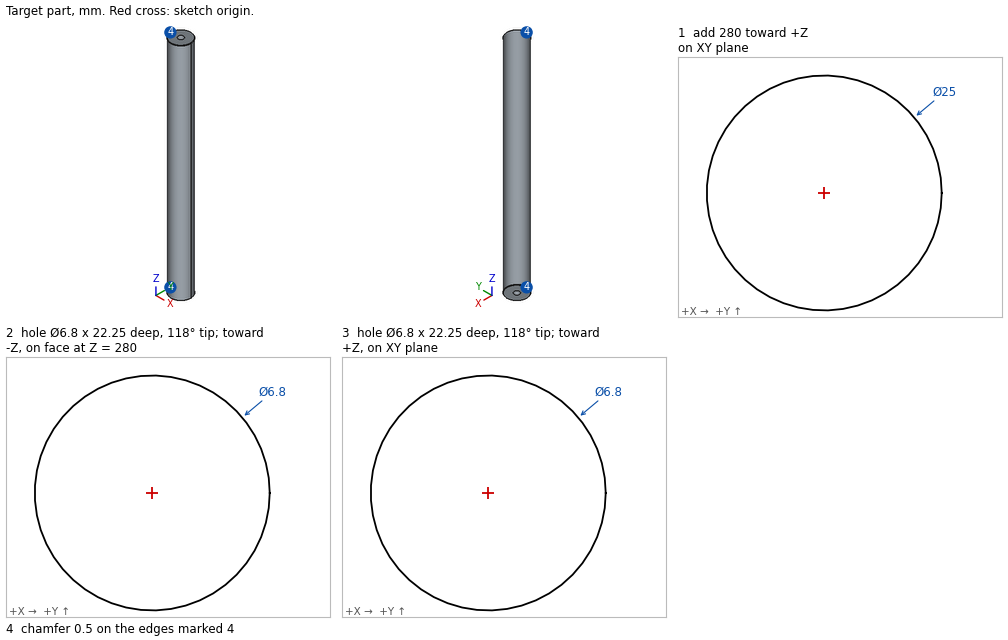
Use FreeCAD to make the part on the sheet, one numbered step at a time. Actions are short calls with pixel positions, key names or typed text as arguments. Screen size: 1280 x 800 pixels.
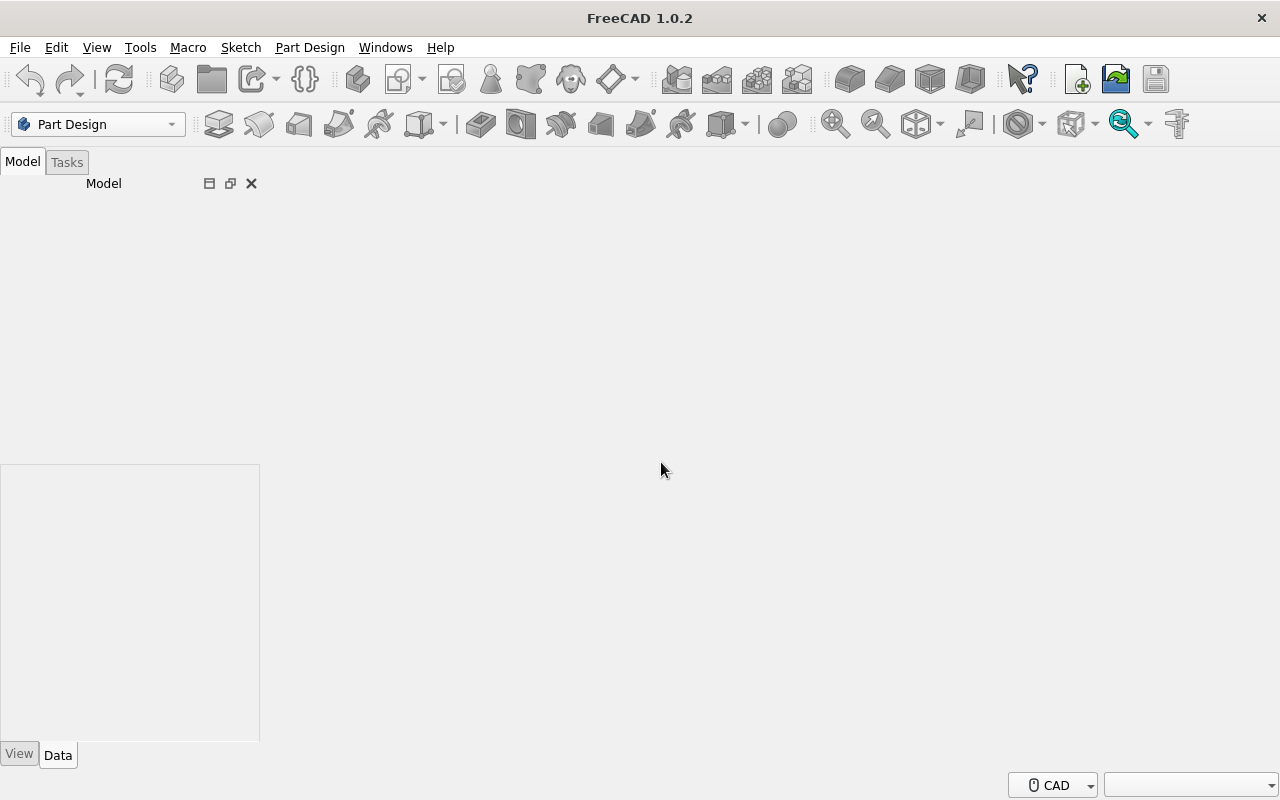
click(1076, 80)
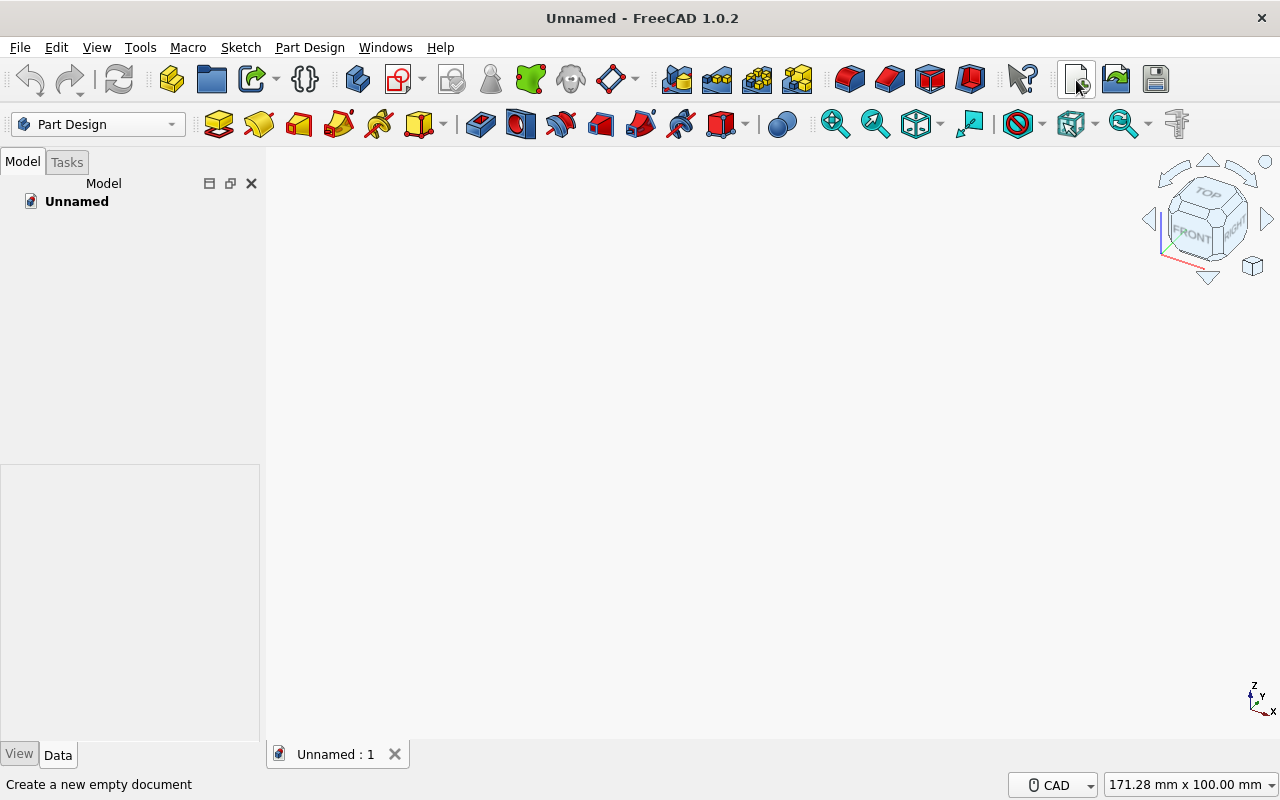
click(398, 80)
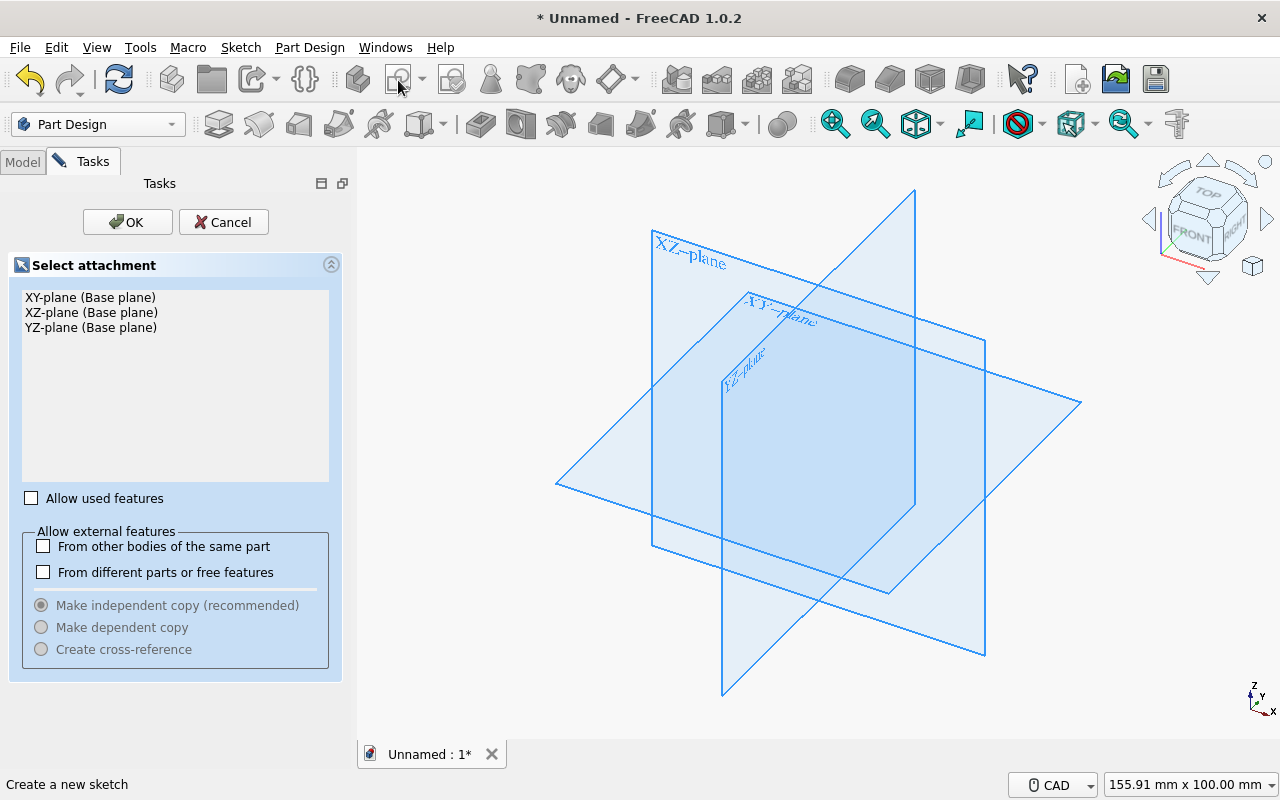
click(82, 298)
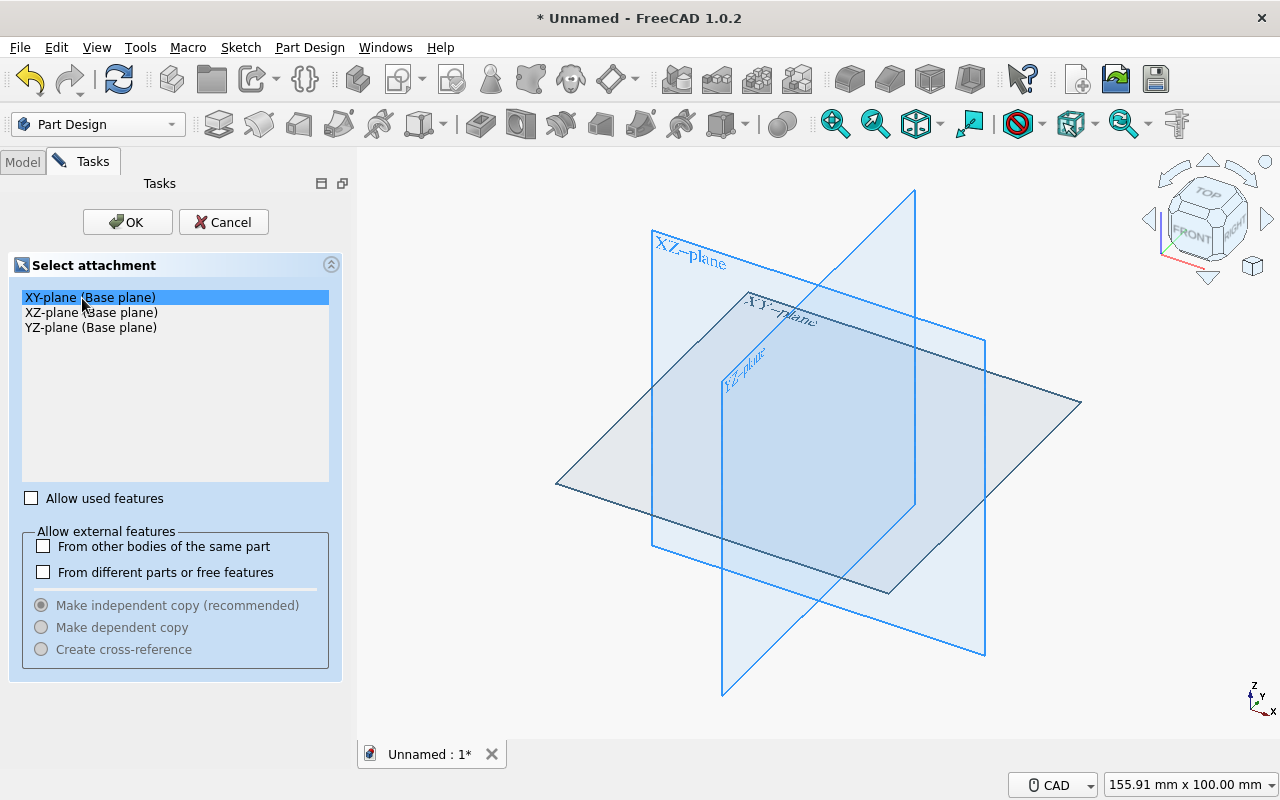
click(128, 222)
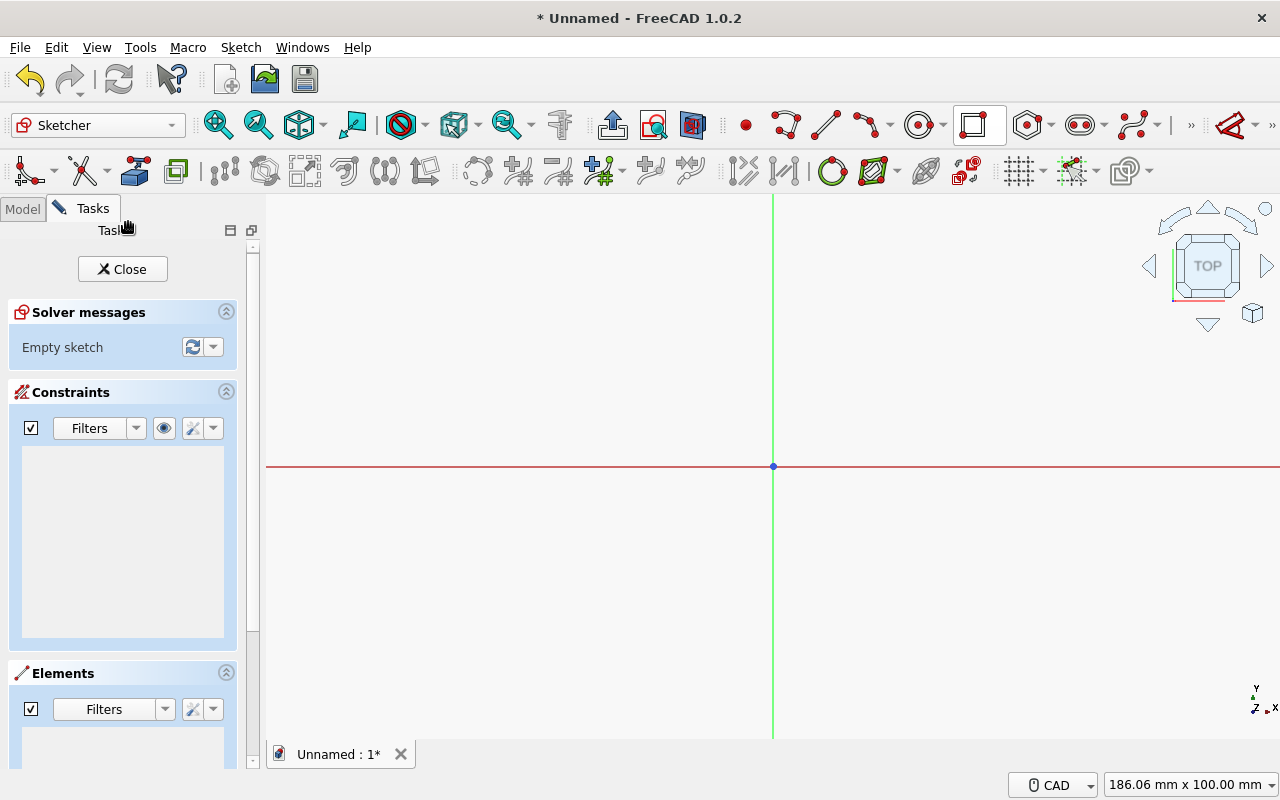
scroll(813, 466, up, 5)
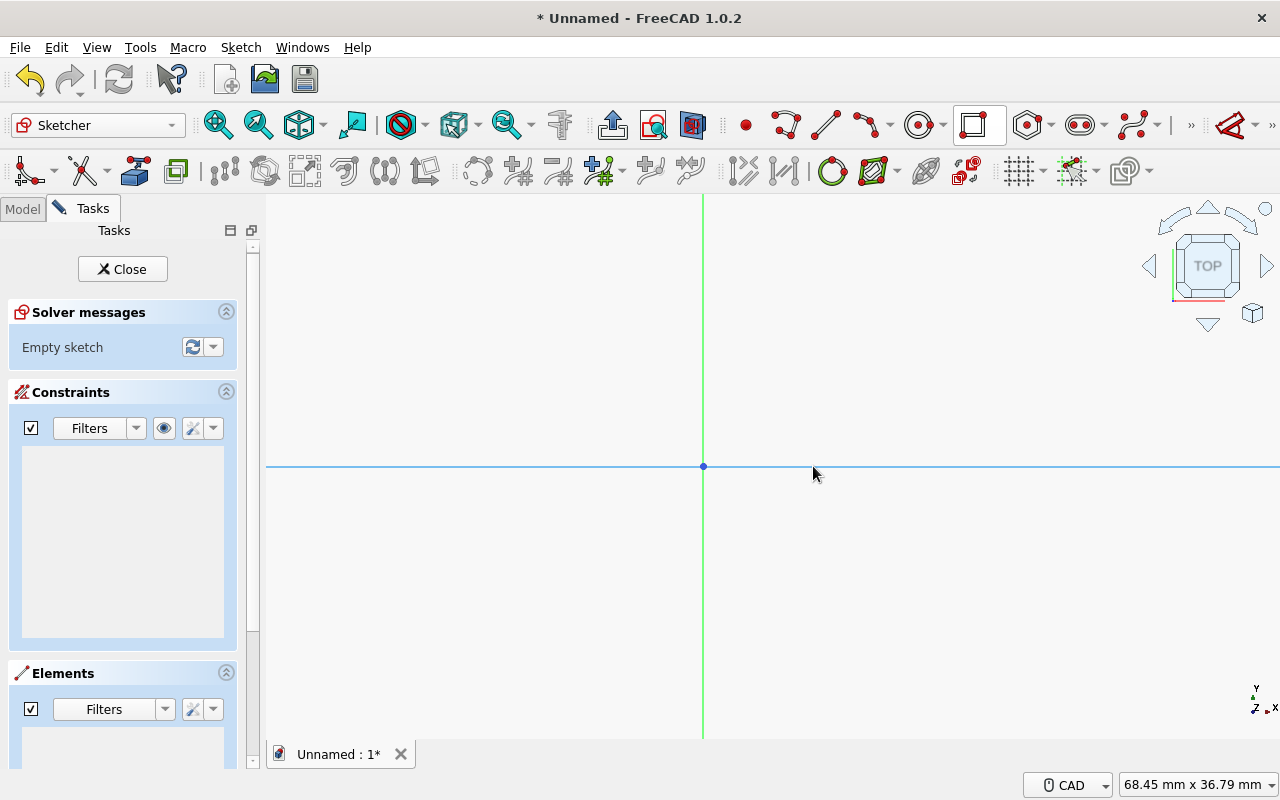
click(920, 126)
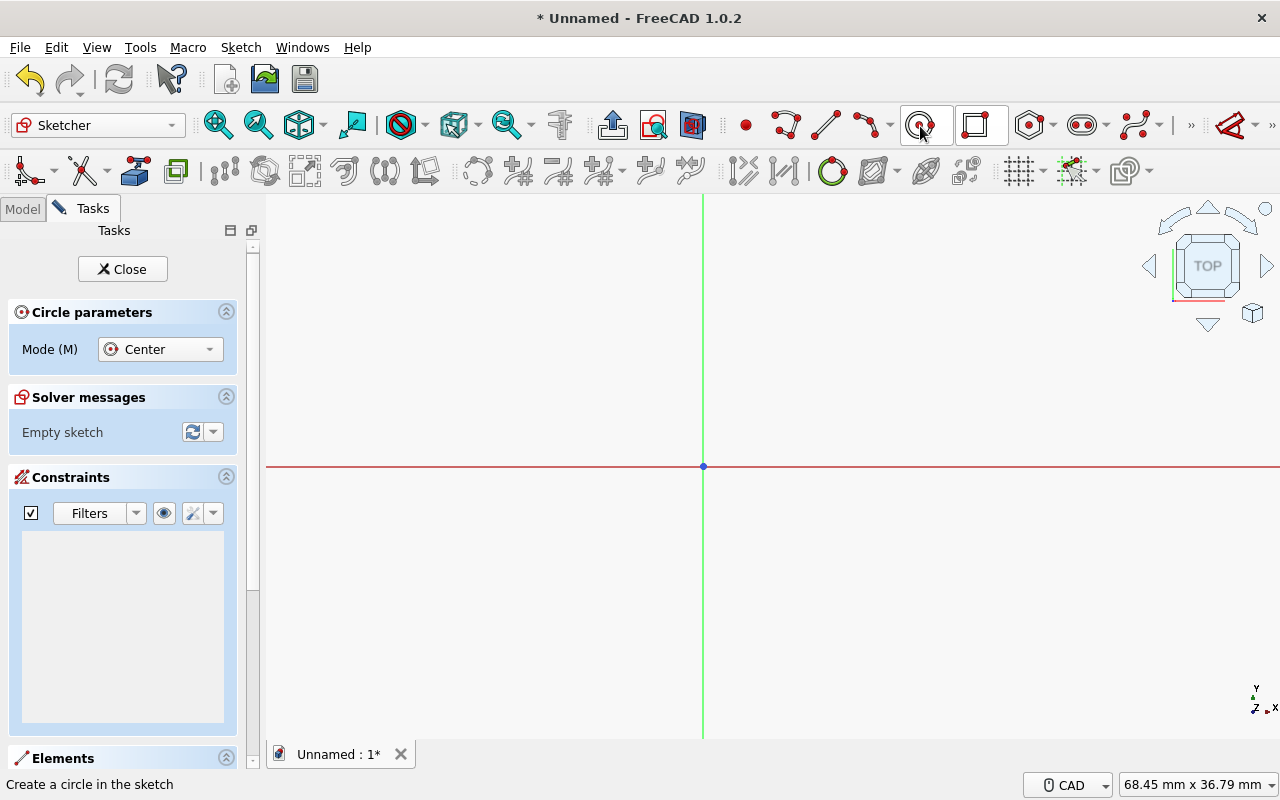
click(703, 466)
click(834, 336)
key(Escape)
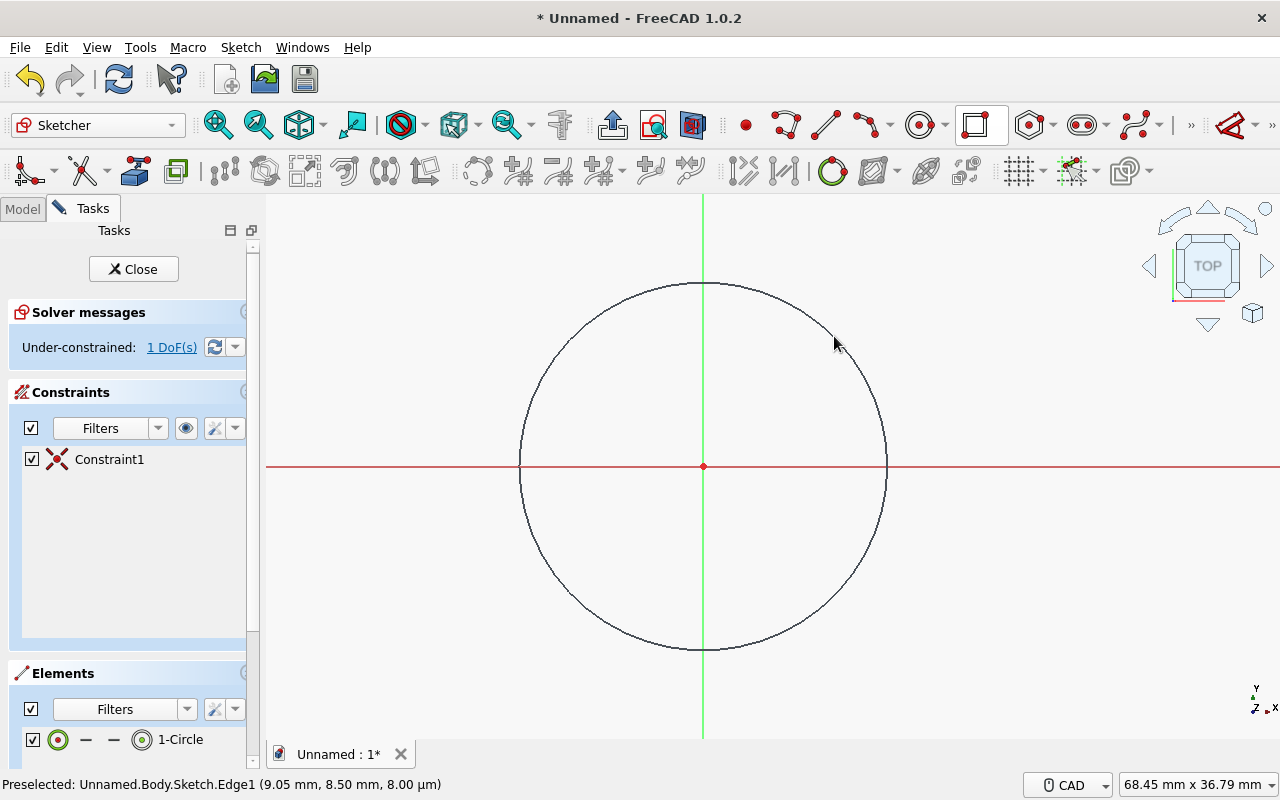
click(1230, 126)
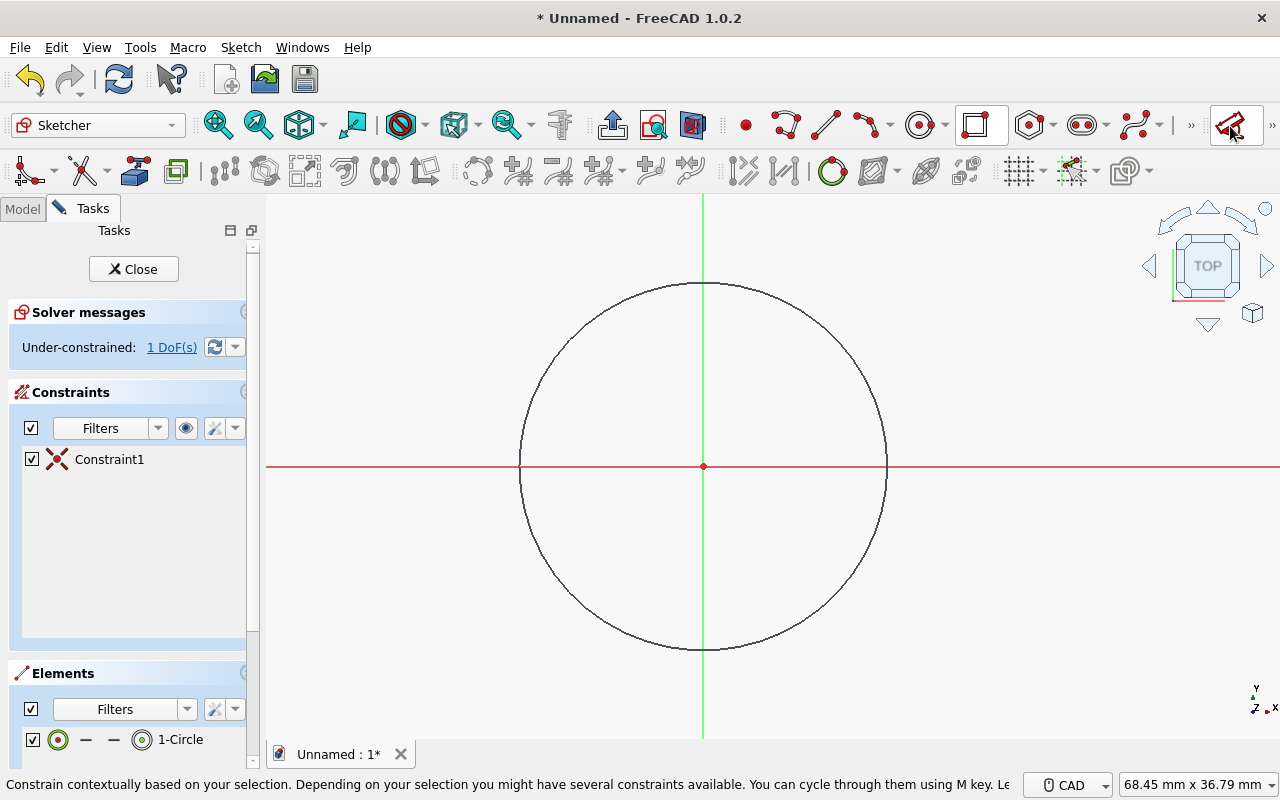
click(833, 336)
click(856, 313)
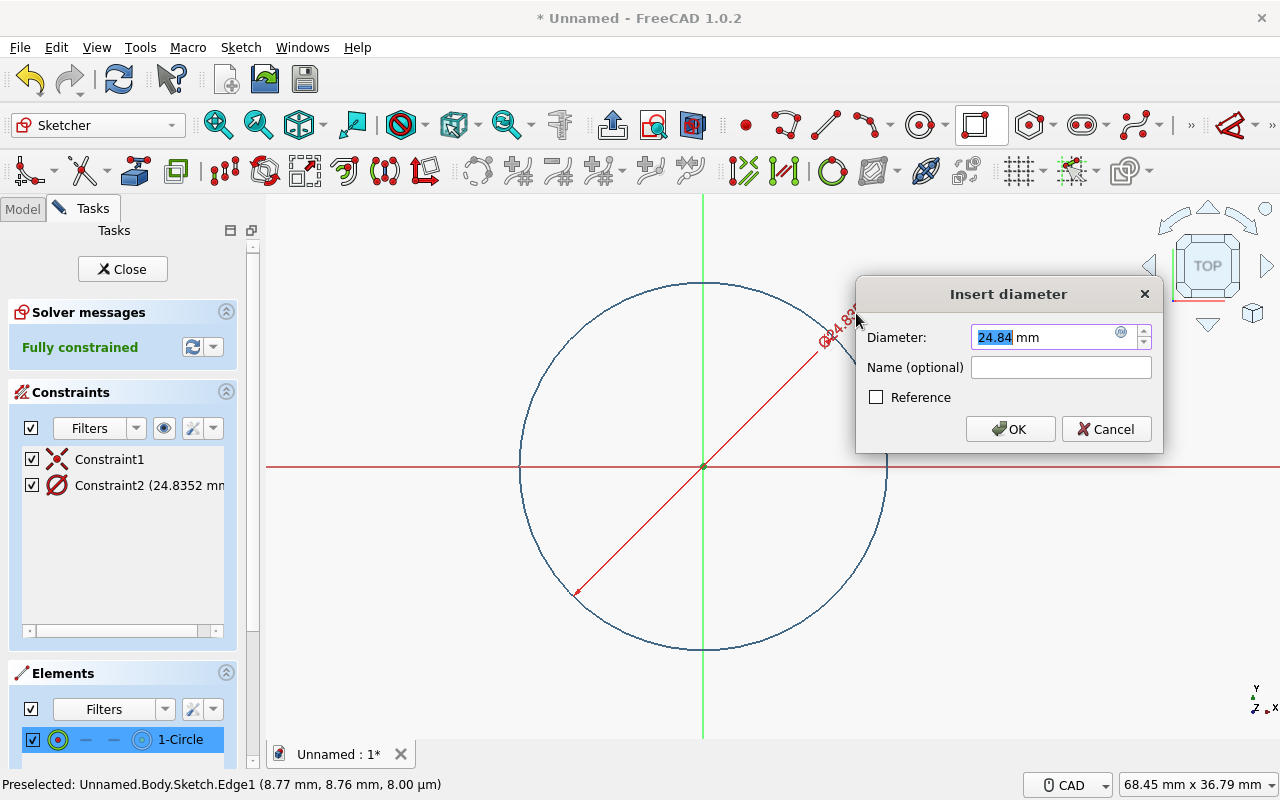
text(25)
key(Return)
key(Escape)